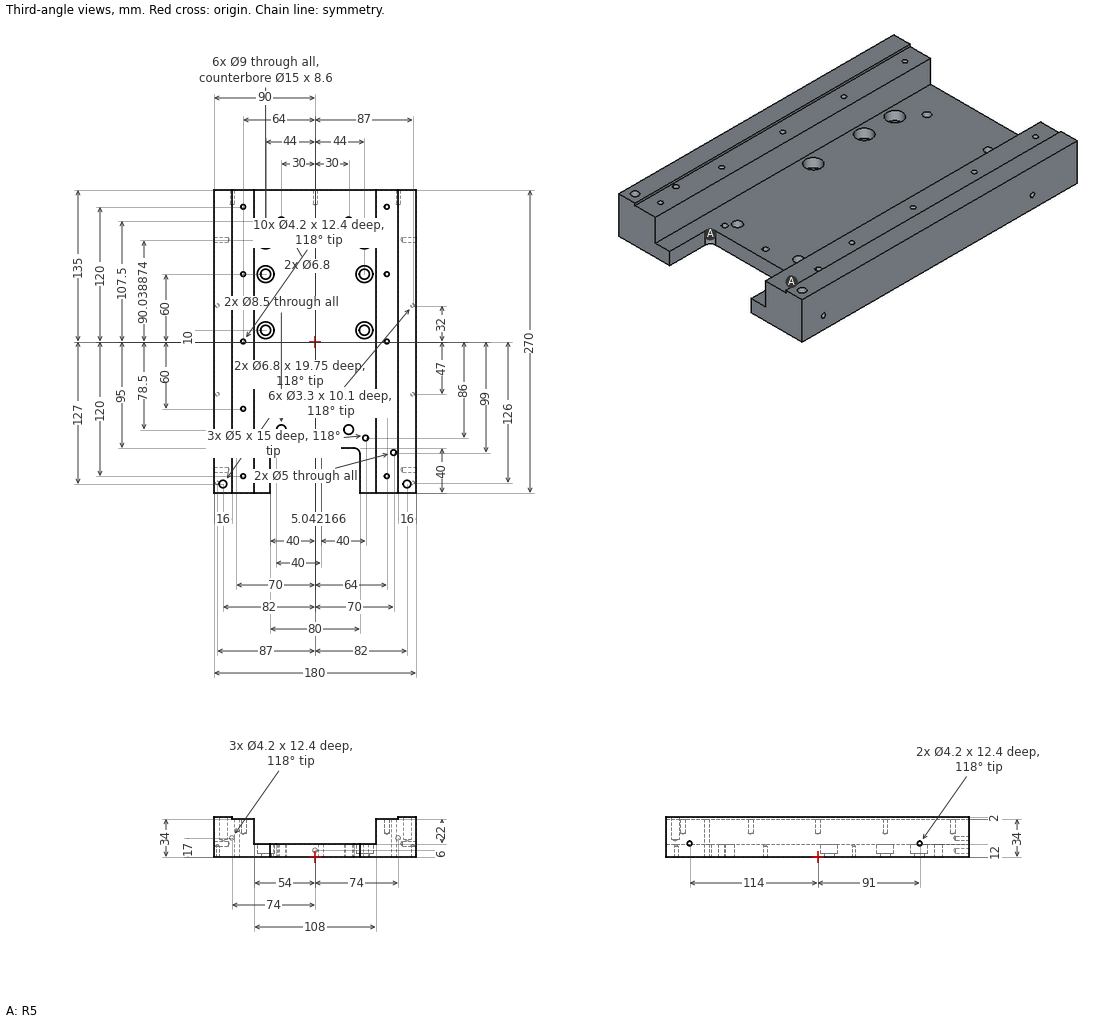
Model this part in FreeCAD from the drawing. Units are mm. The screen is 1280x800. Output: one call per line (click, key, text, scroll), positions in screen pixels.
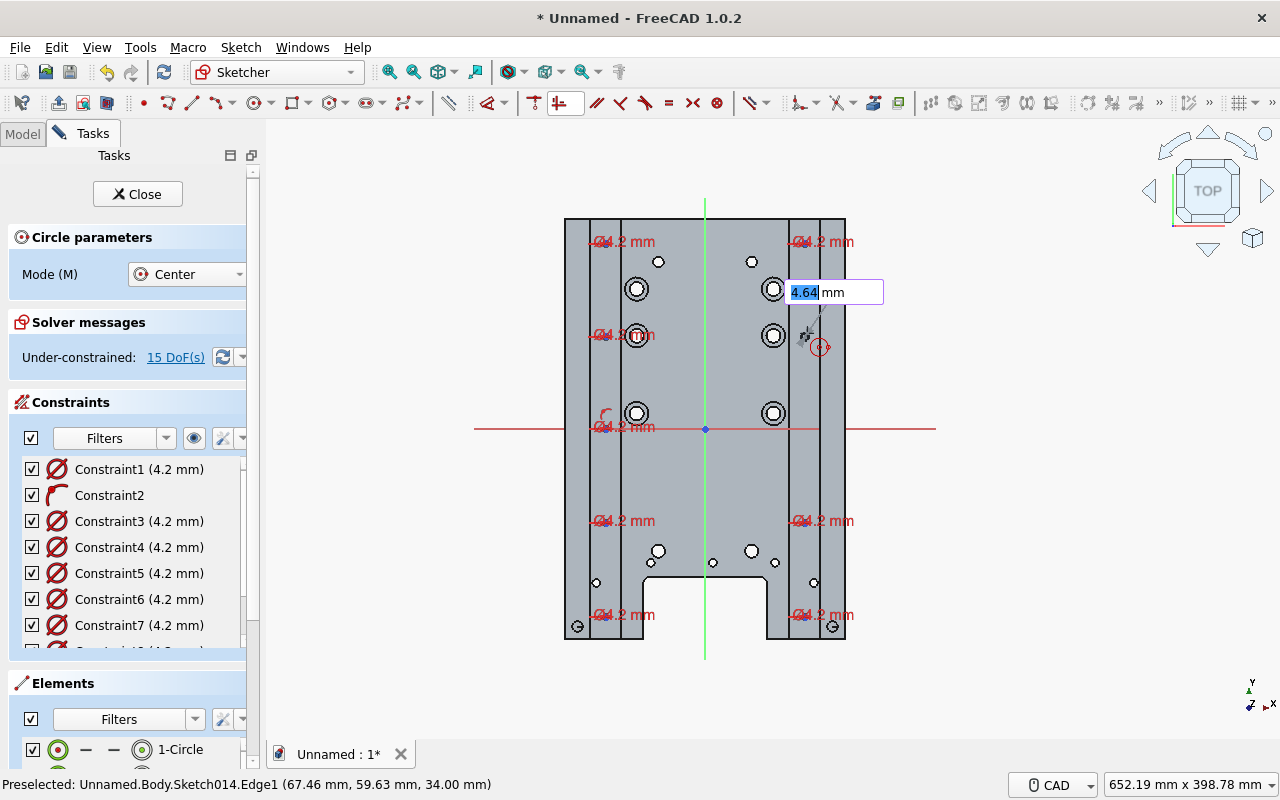
text(4.2)
key(Return)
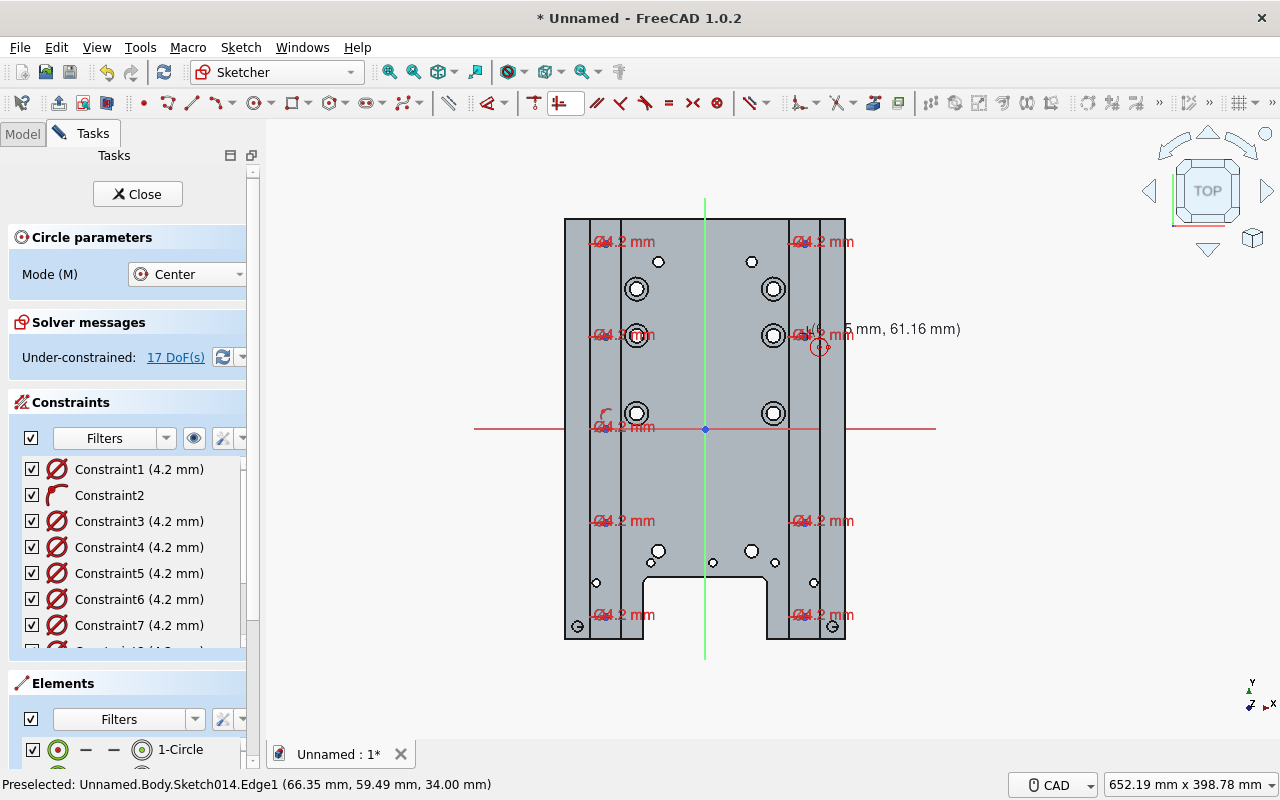
scroll(805, 429, up, 10)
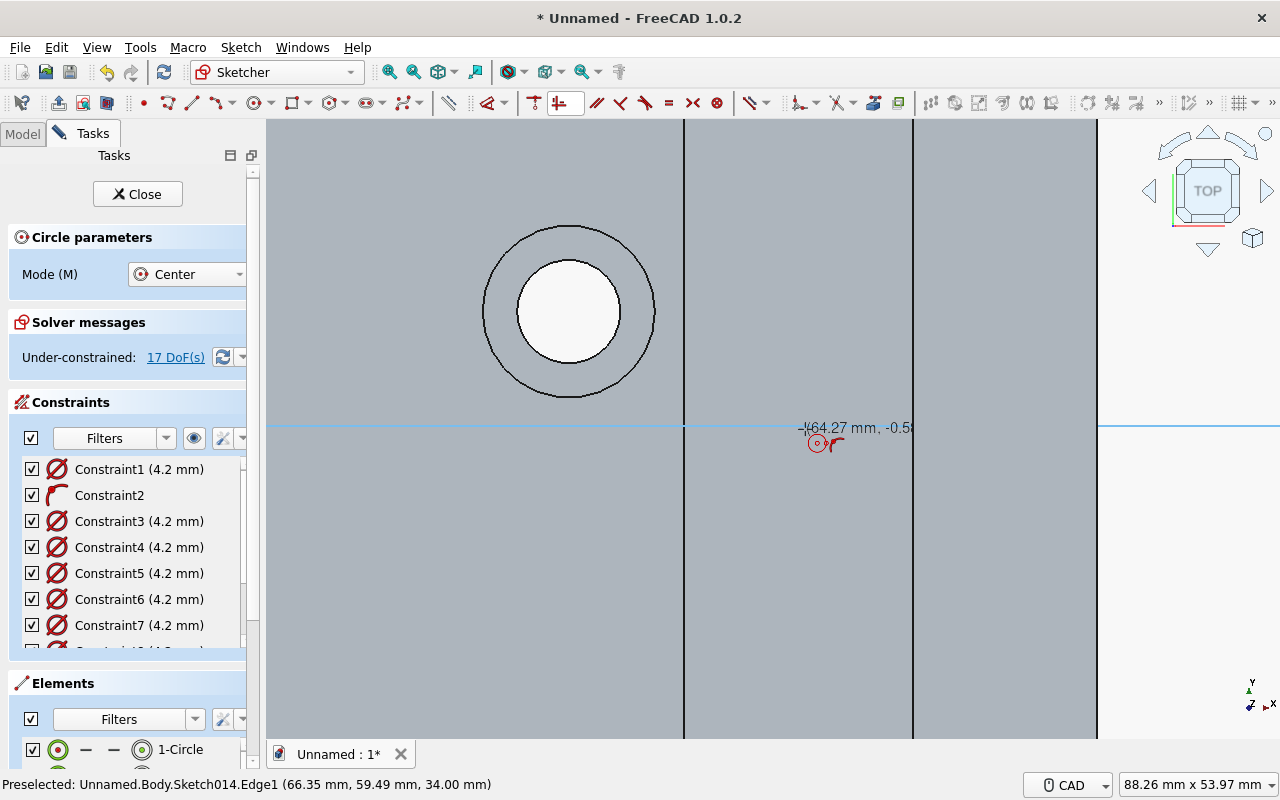
scroll(805, 429, down, 10)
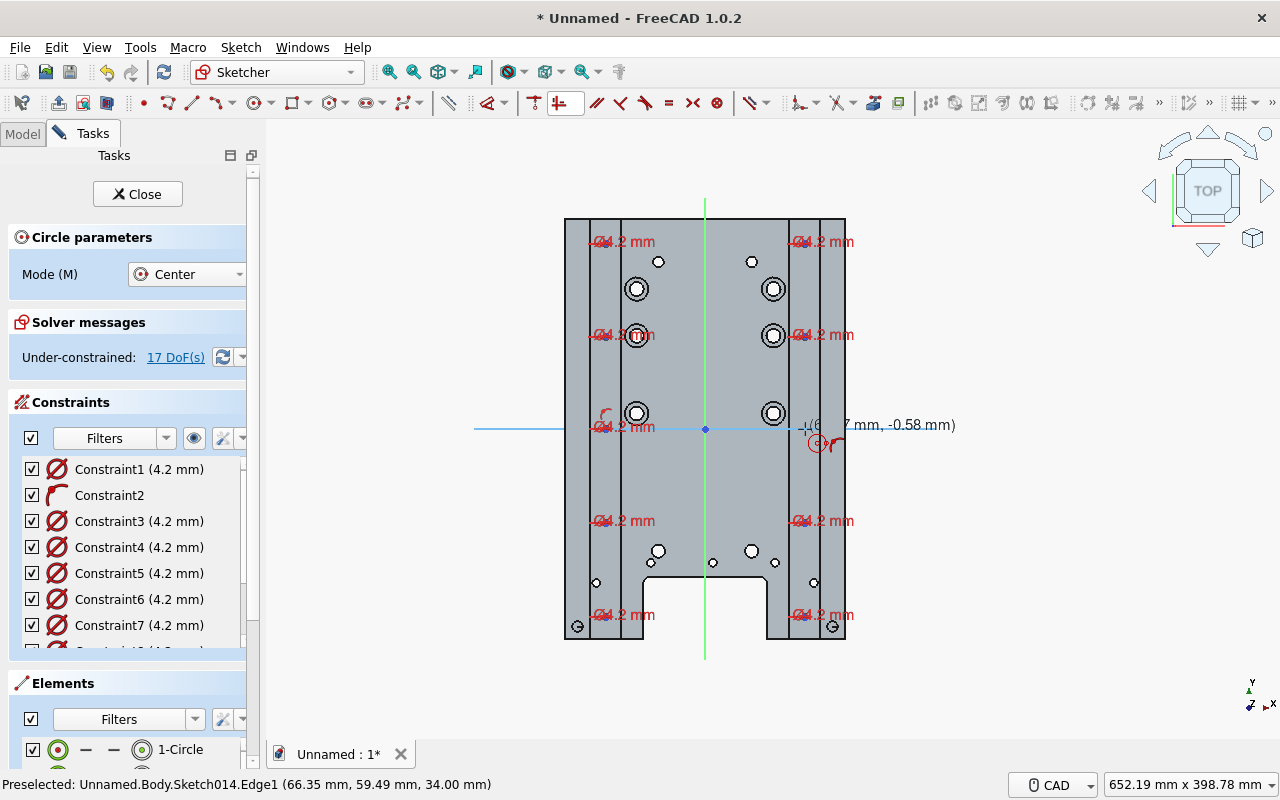
click(805, 429)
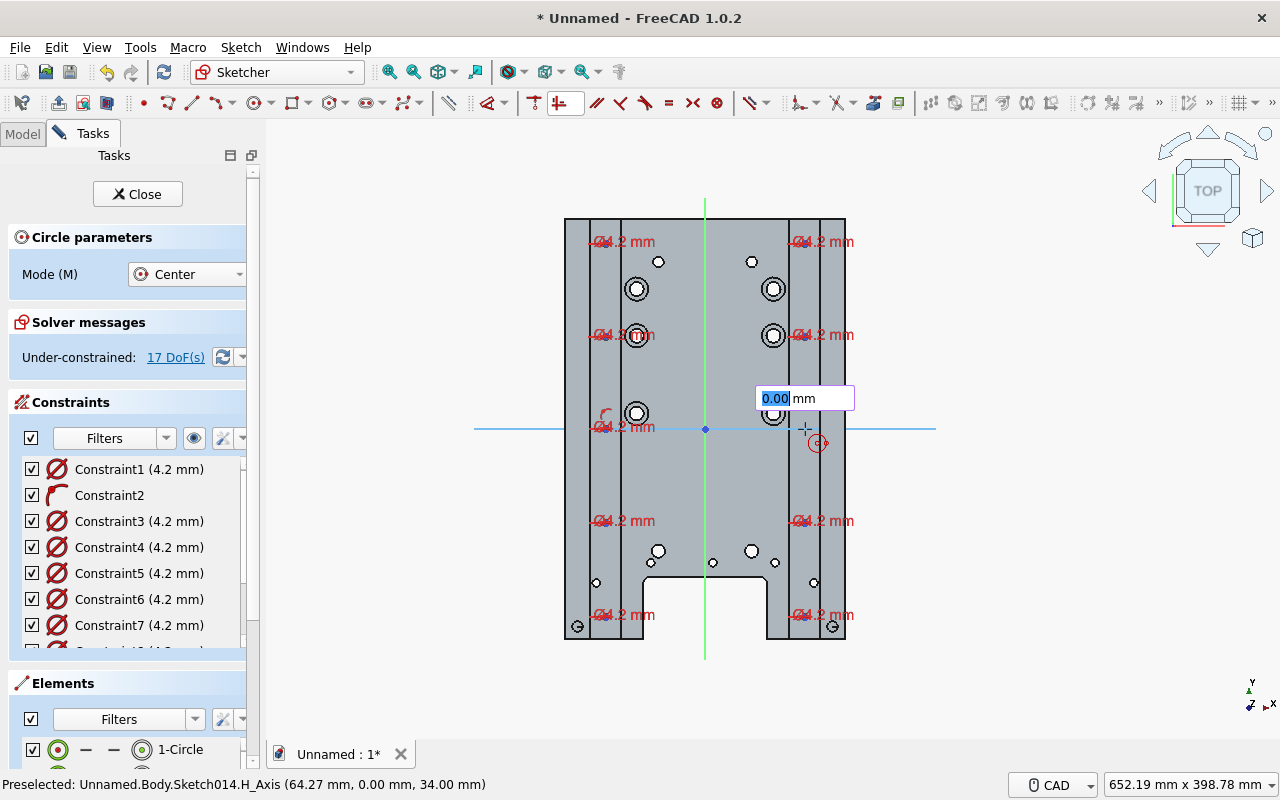
scroll(803, 432, up, 9)
move(803, 430)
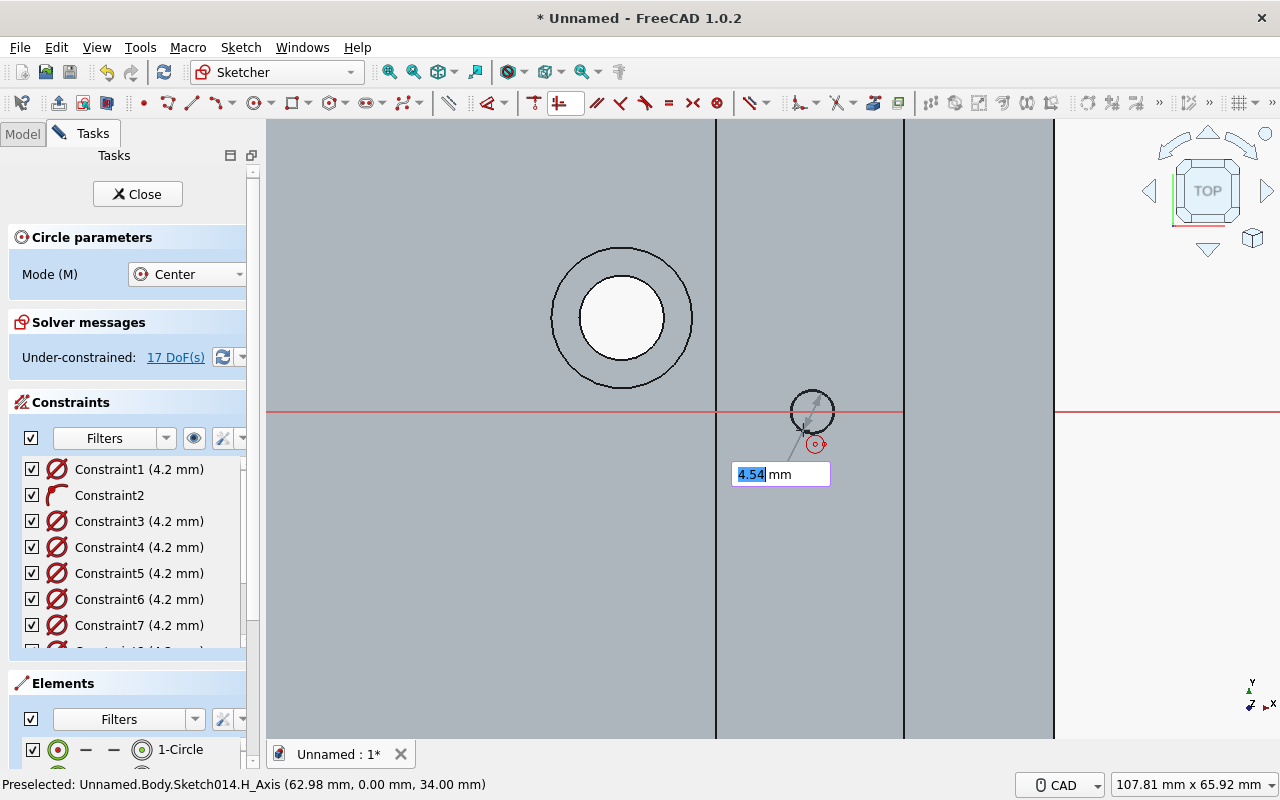
text(4.2)
key(Return)
key(Escape)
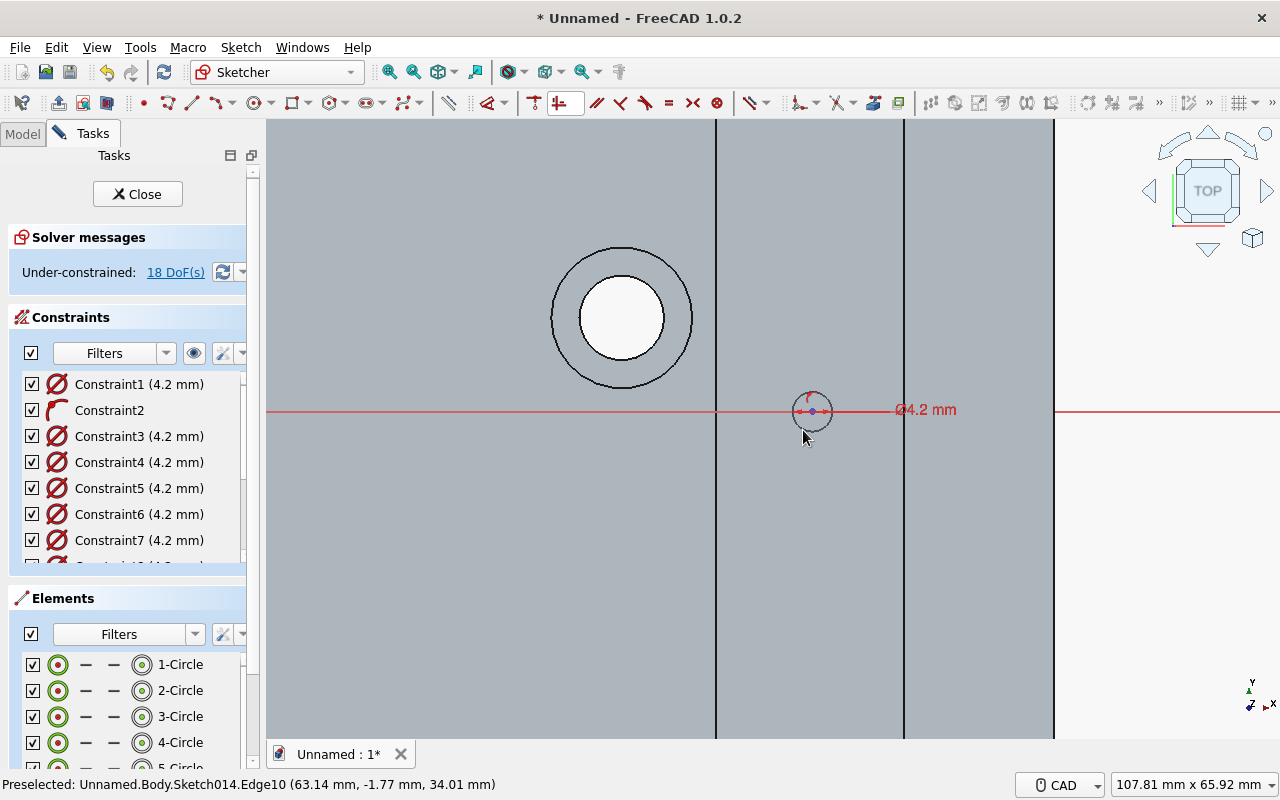
scroll(803, 432, down, 9)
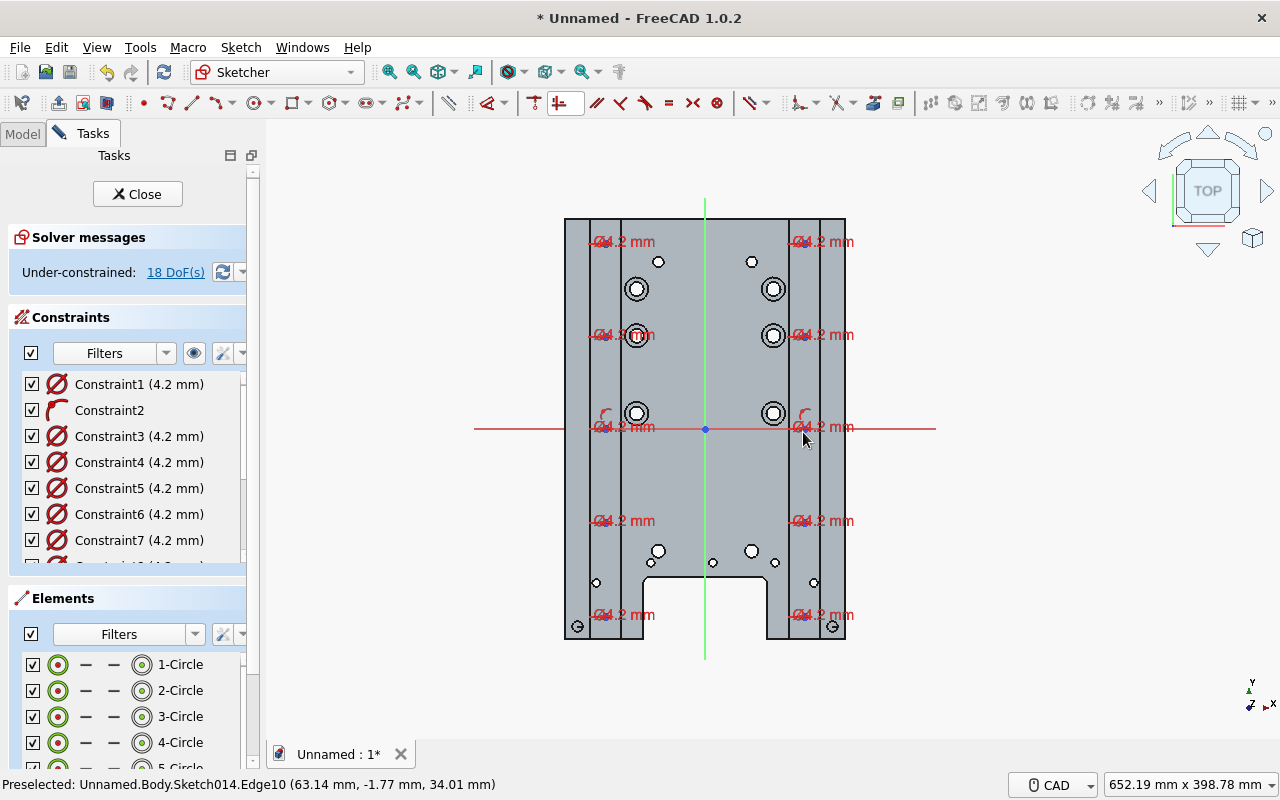
click(606, 429)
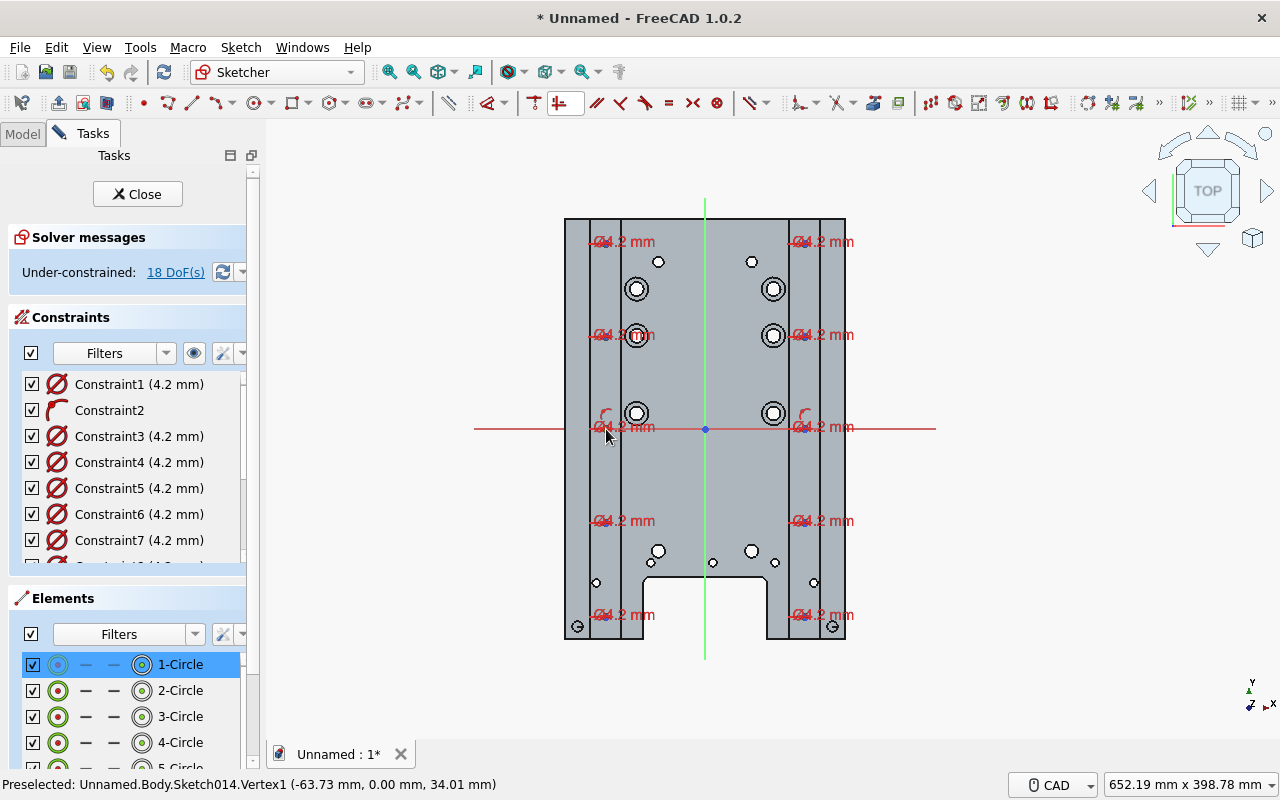
click(606, 337)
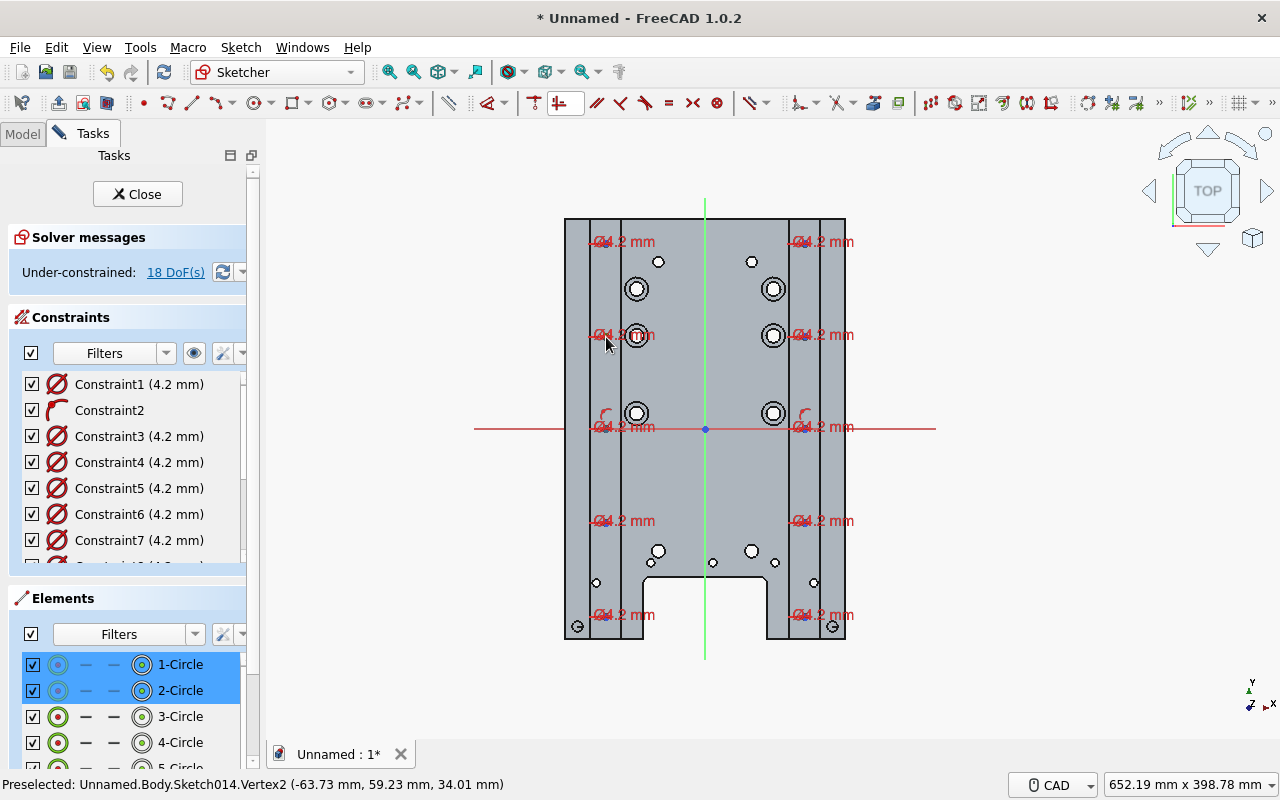
click(578, 104)